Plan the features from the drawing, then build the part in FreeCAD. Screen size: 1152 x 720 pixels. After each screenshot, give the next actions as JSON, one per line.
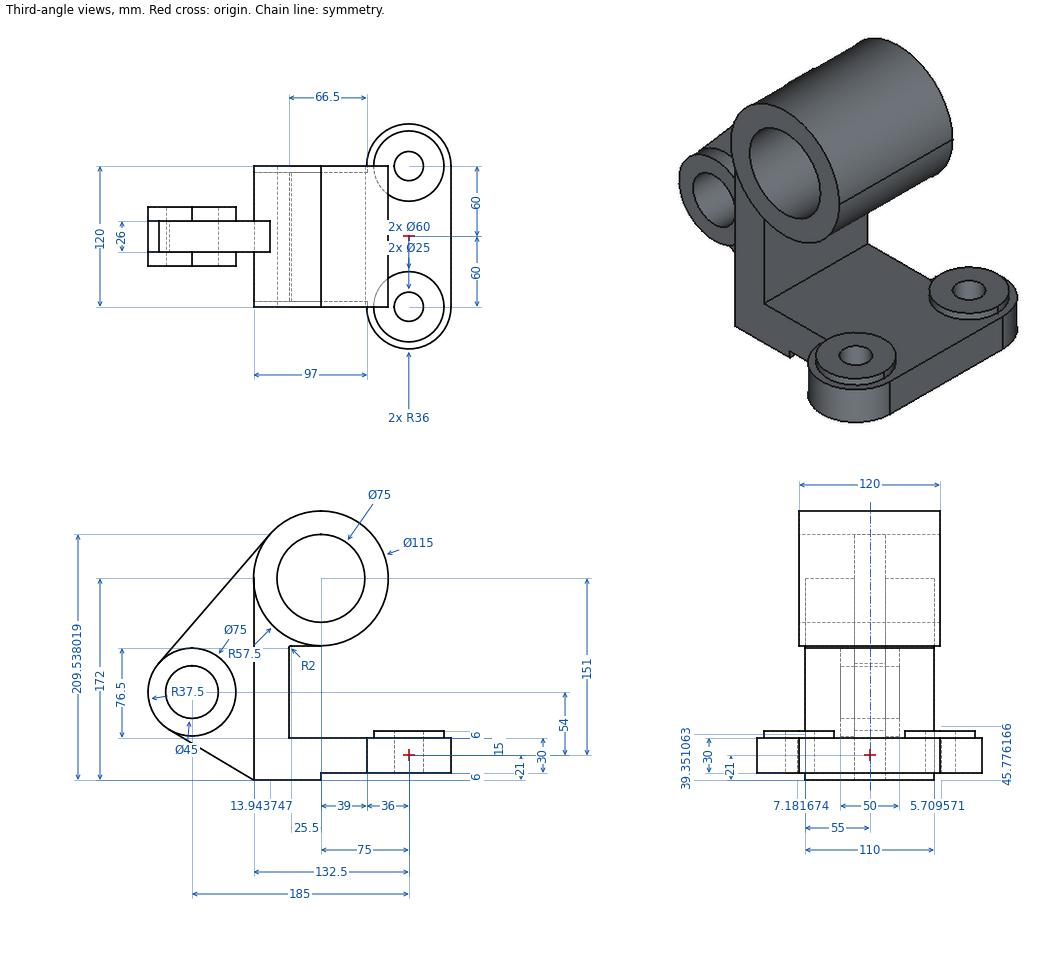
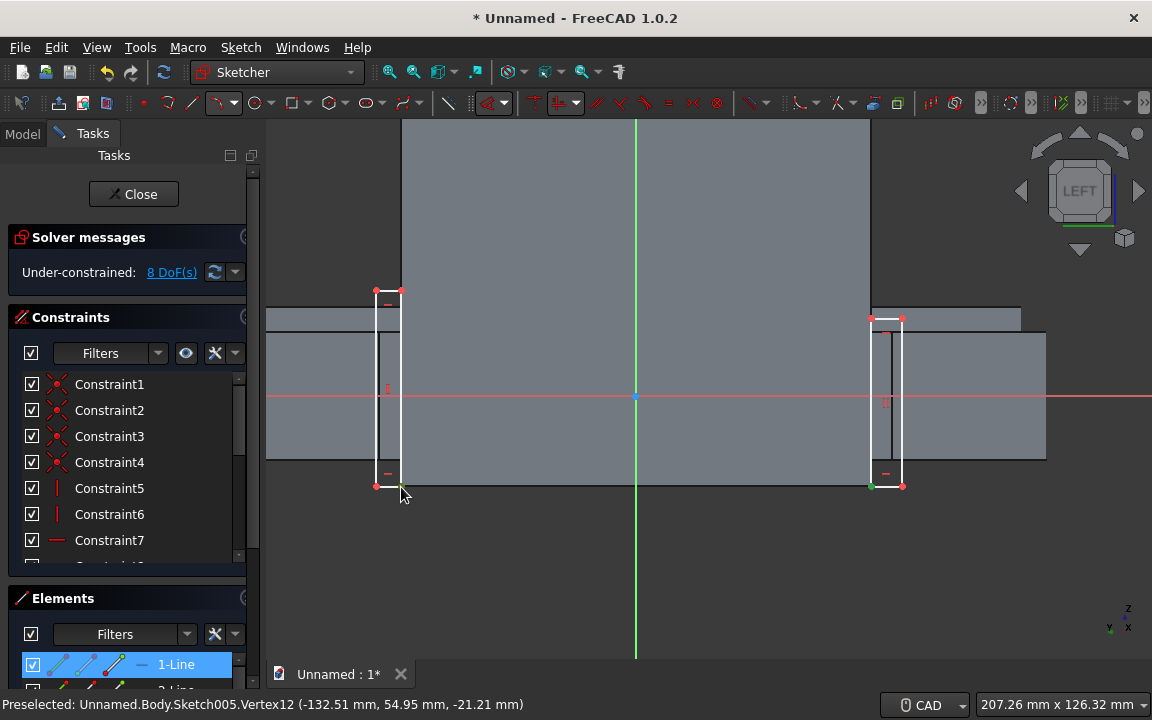
{"action": "left_click", "coordinate": [636, 596]}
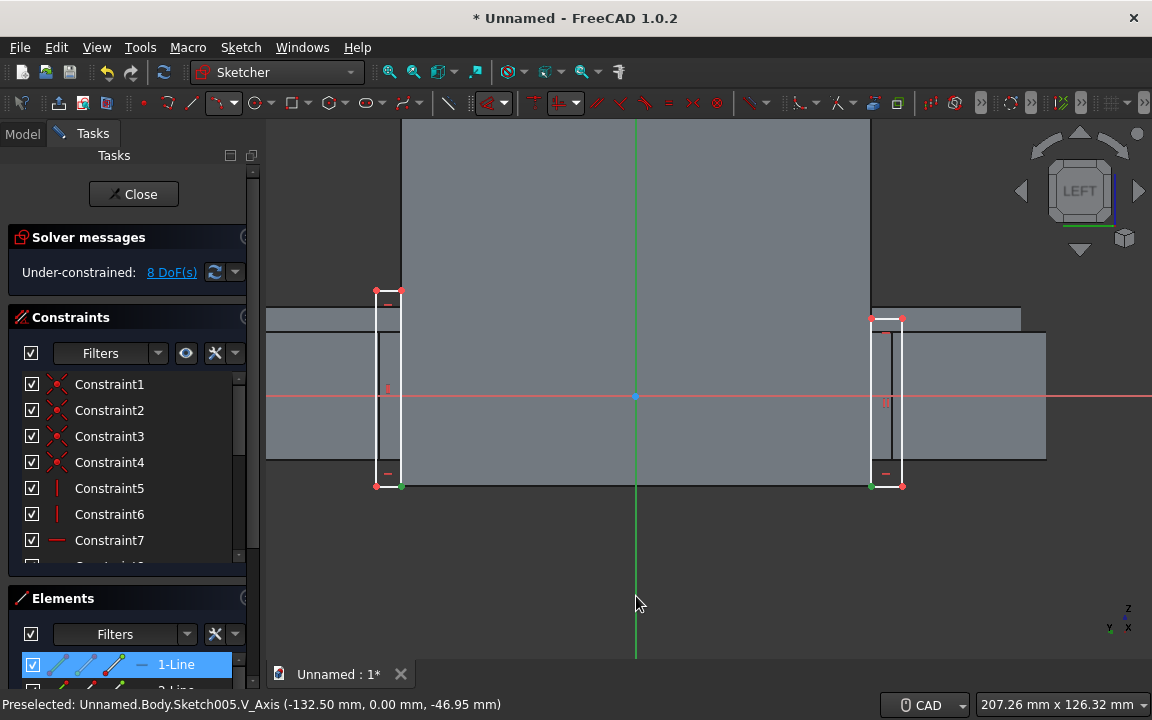
{"action": "key", "text": "s"}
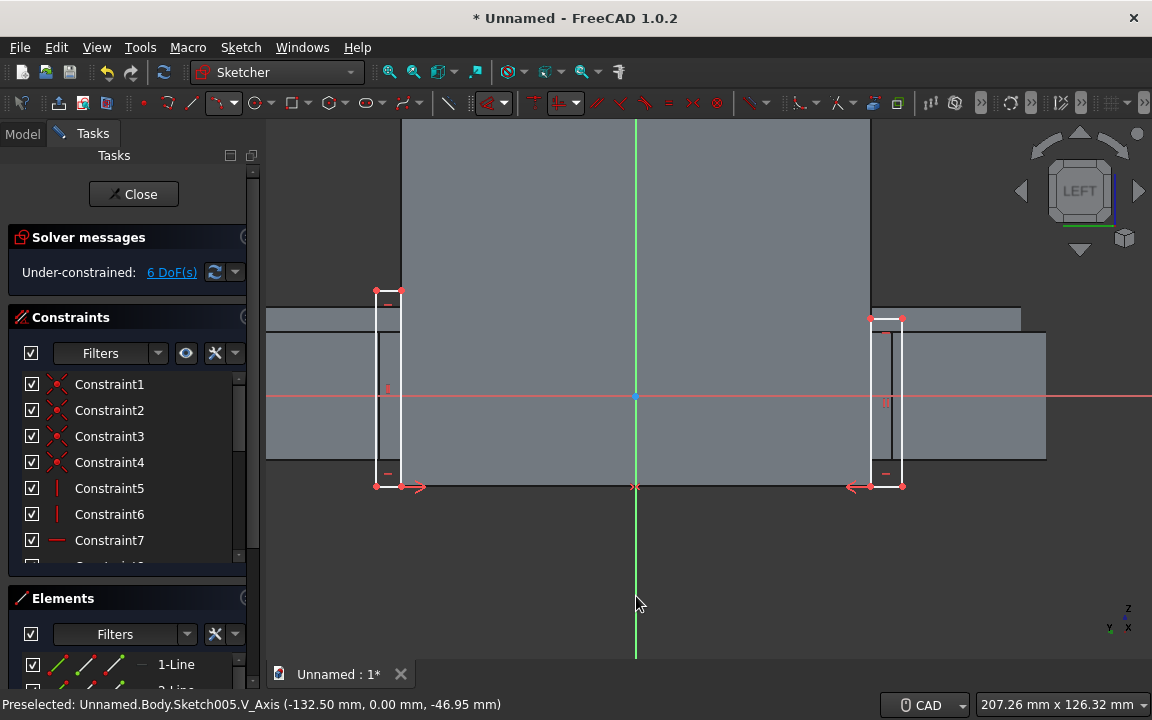
{"action": "left_click", "coordinate": [871, 319]}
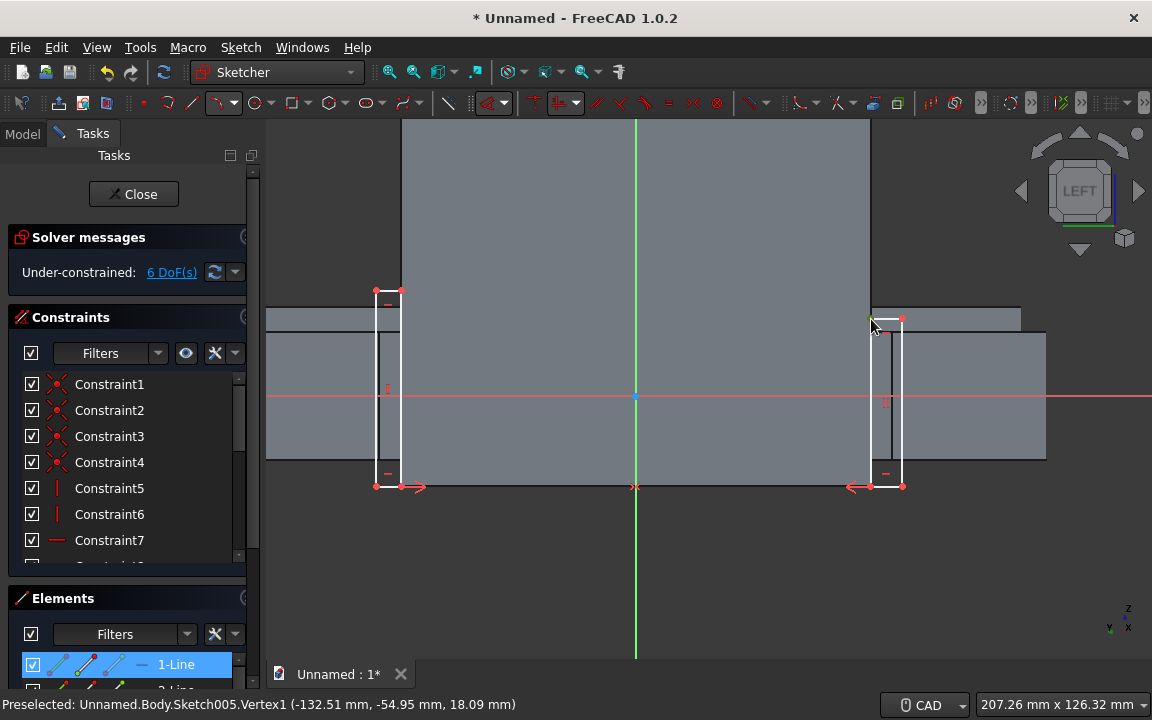
{"action": "left_click", "coordinate": [506, 104]}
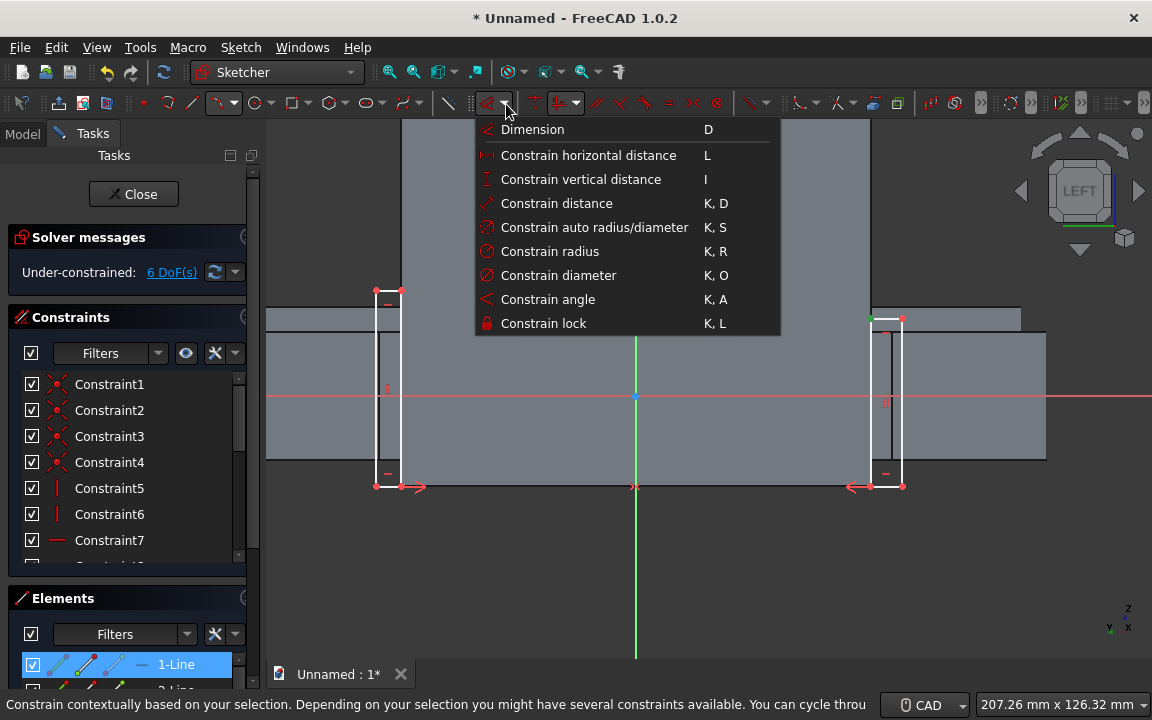
{"action": "left_click", "coordinate": [628, 155]}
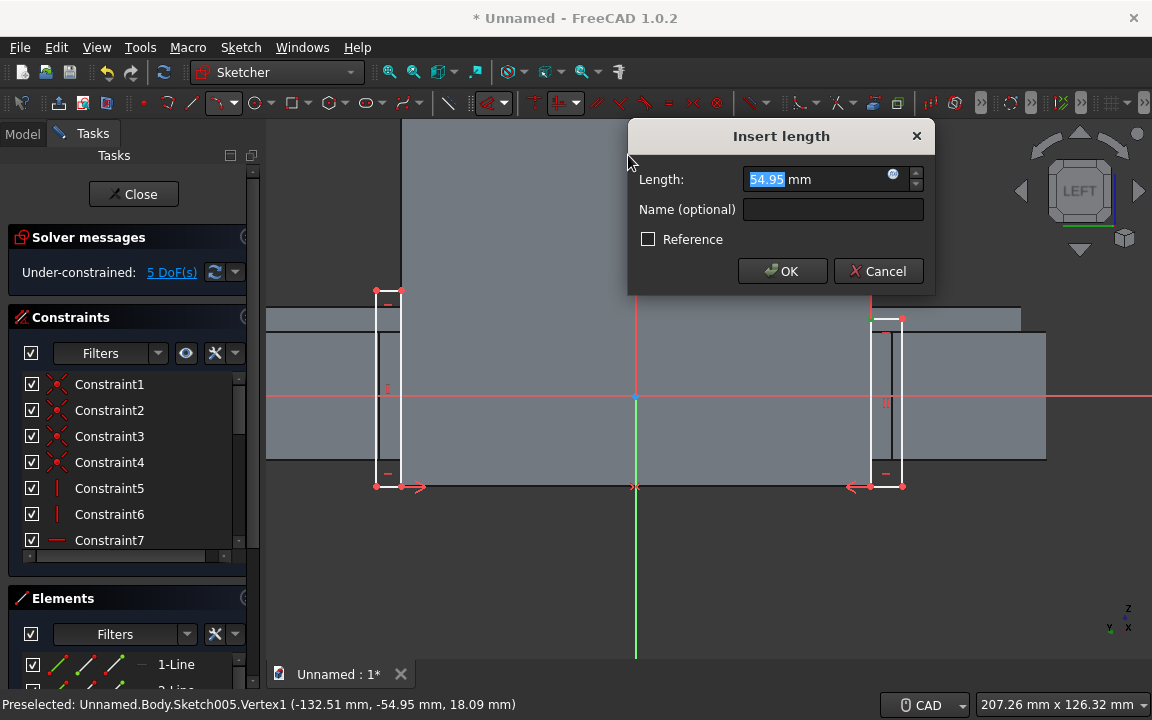
{"action": "type", "text": "55"}
{"action": "key", "text": "Return"}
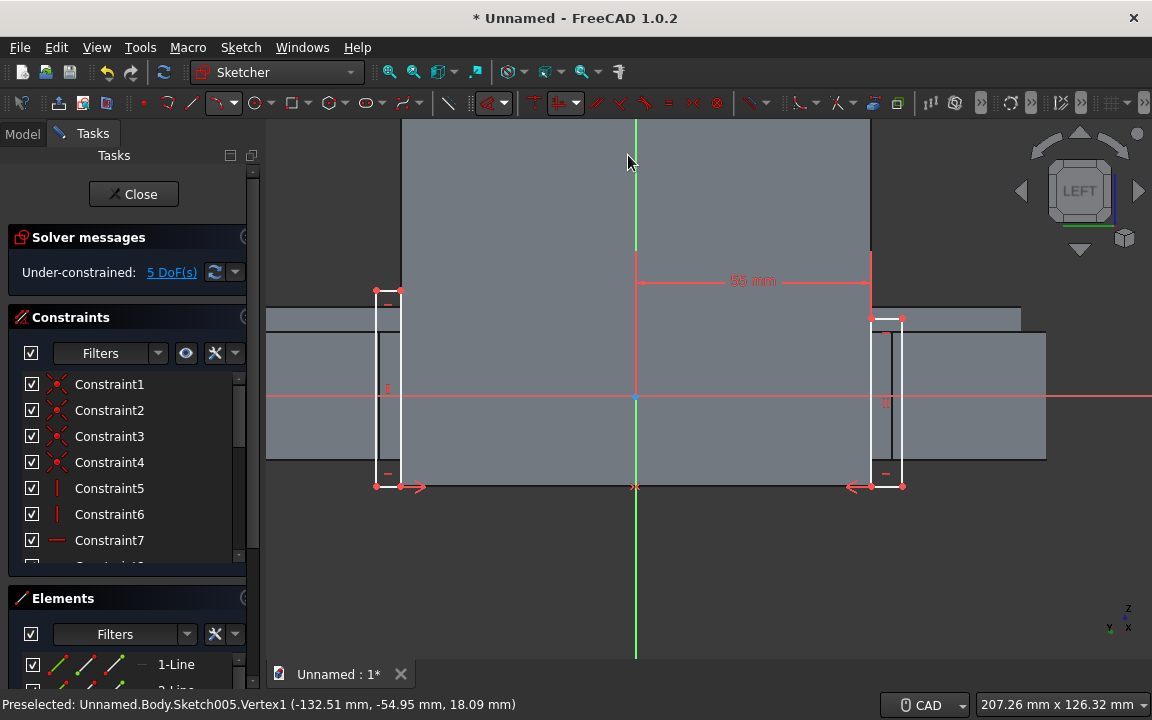
{"action": "left_click", "coordinate": [871, 487]}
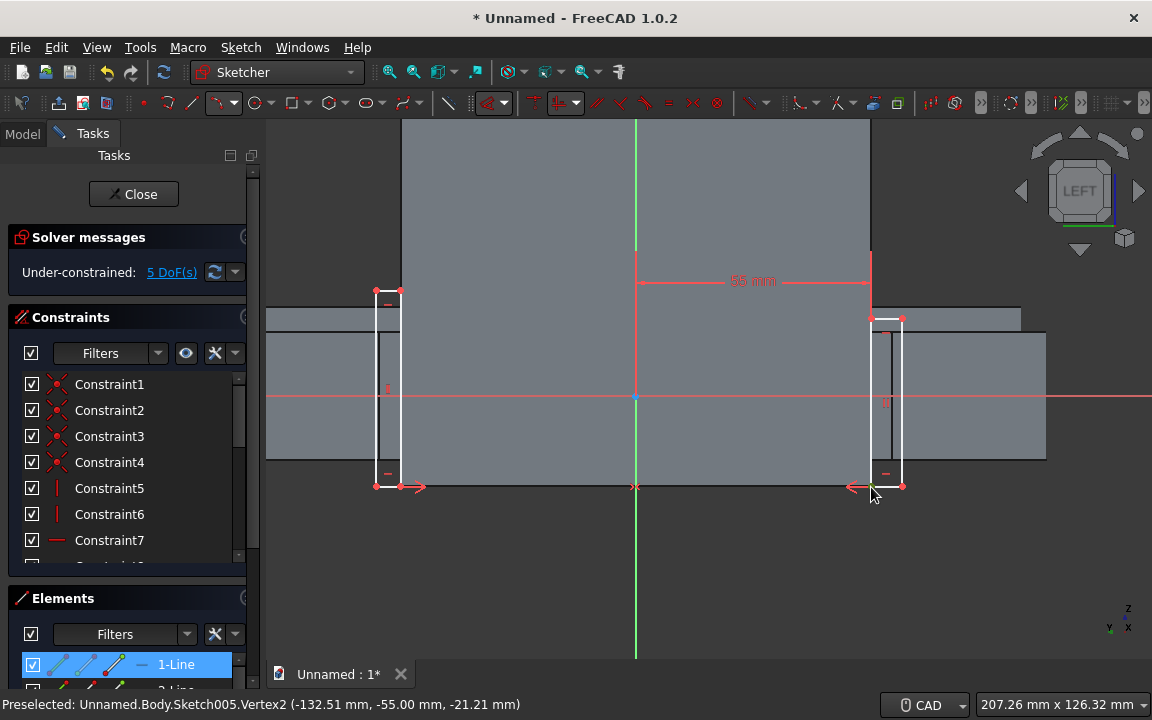
{"action": "key", "text": "i"}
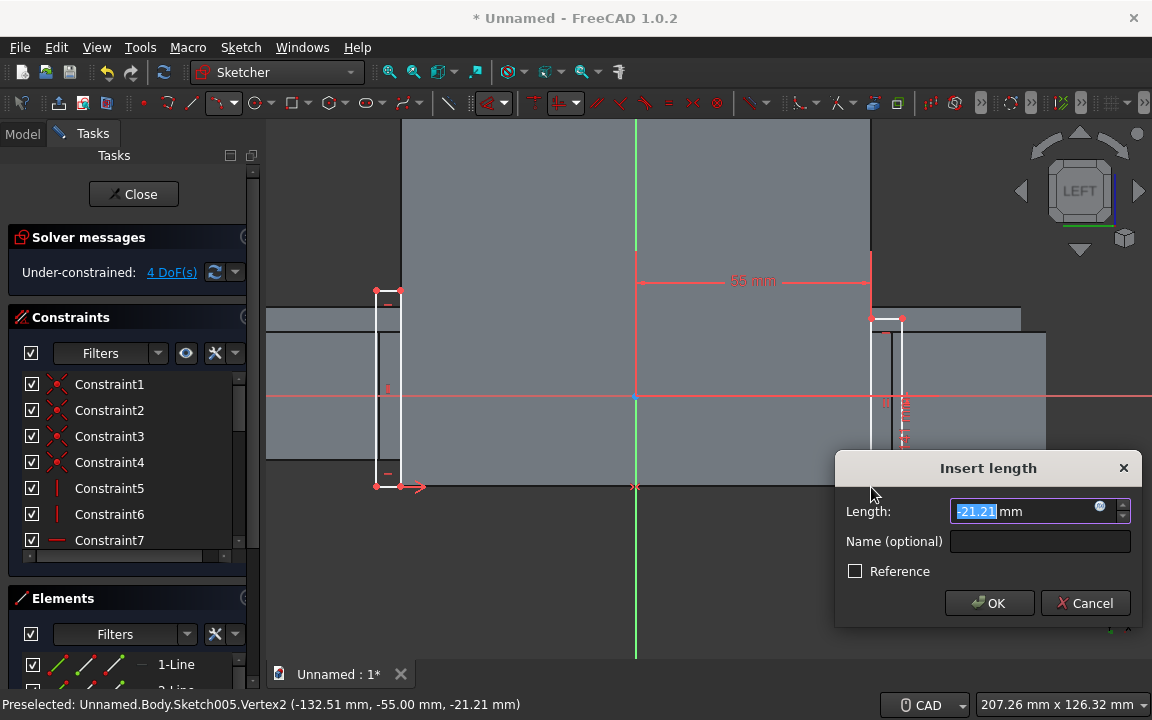
{"action": "type", "text": "-21"}
{"action": "key", "text": "Return"}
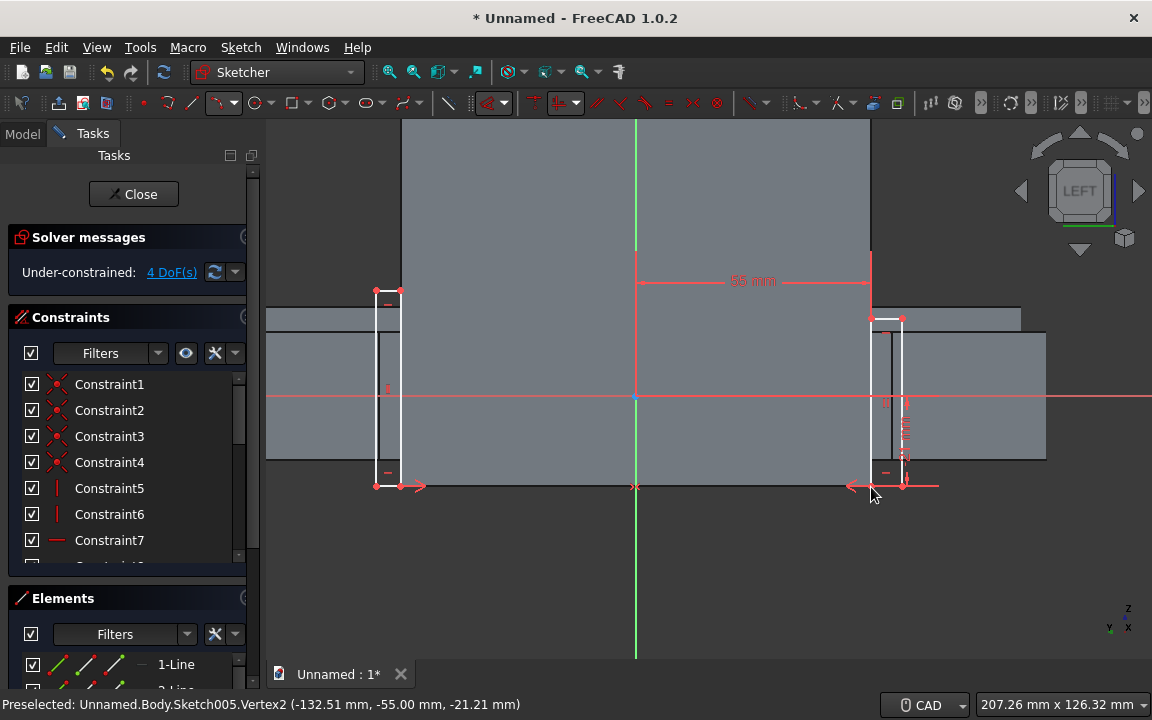
{"action": "scroll", "coordinate": [880, 486], "scroll_direction": "up", "scroll_amount": 2}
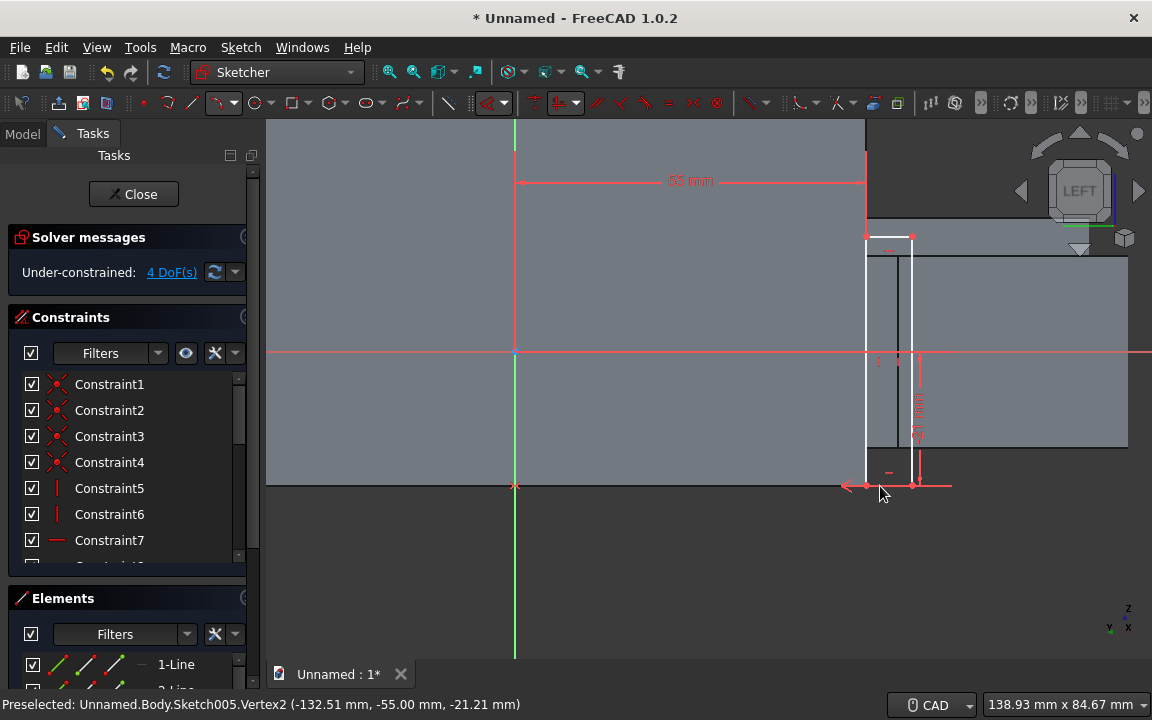
{"action": "left_click", "coordinate": [880, 486]}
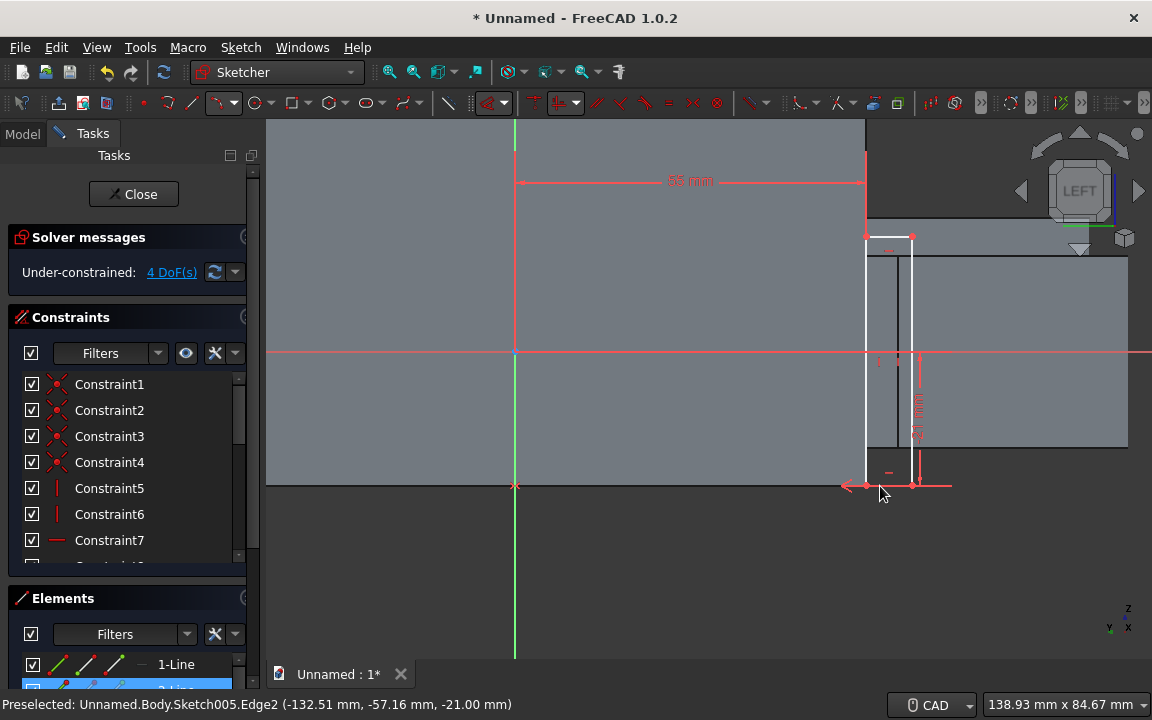
{"action": "key", "text": "l"}